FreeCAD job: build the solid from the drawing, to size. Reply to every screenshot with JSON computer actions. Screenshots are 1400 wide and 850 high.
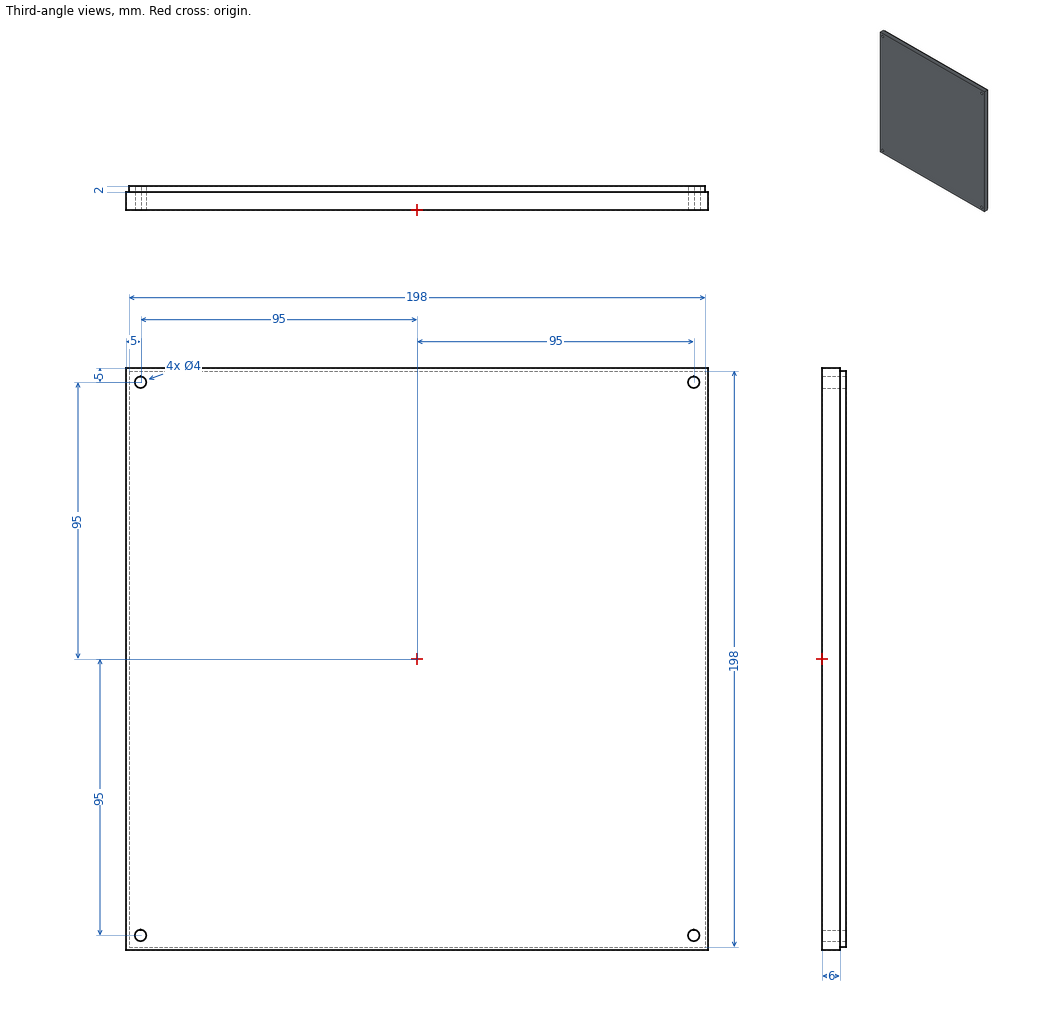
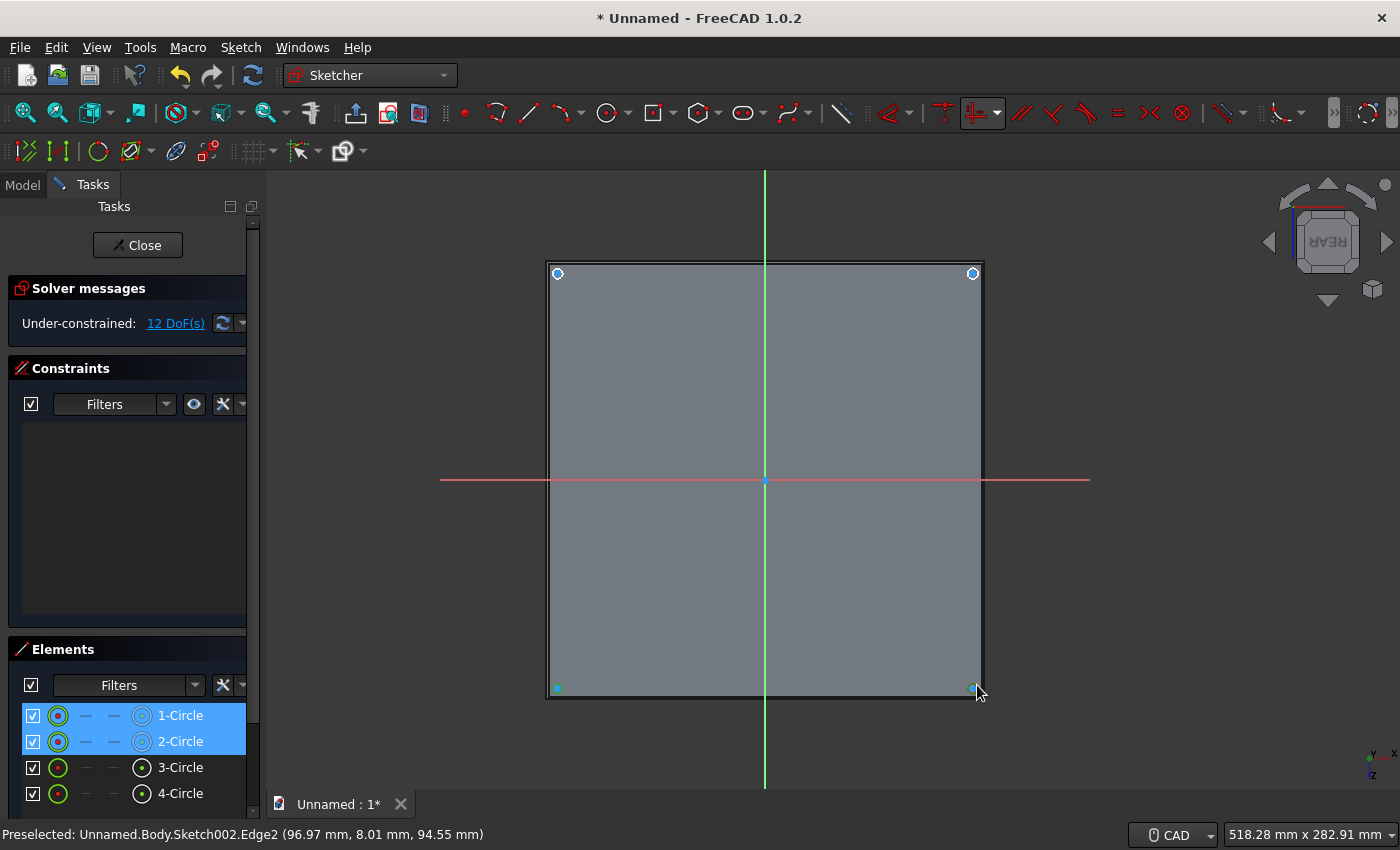
{"action": "scroll", "coordinate": [977, 270], "scroll_direction": "up", "scroll_amount": 5}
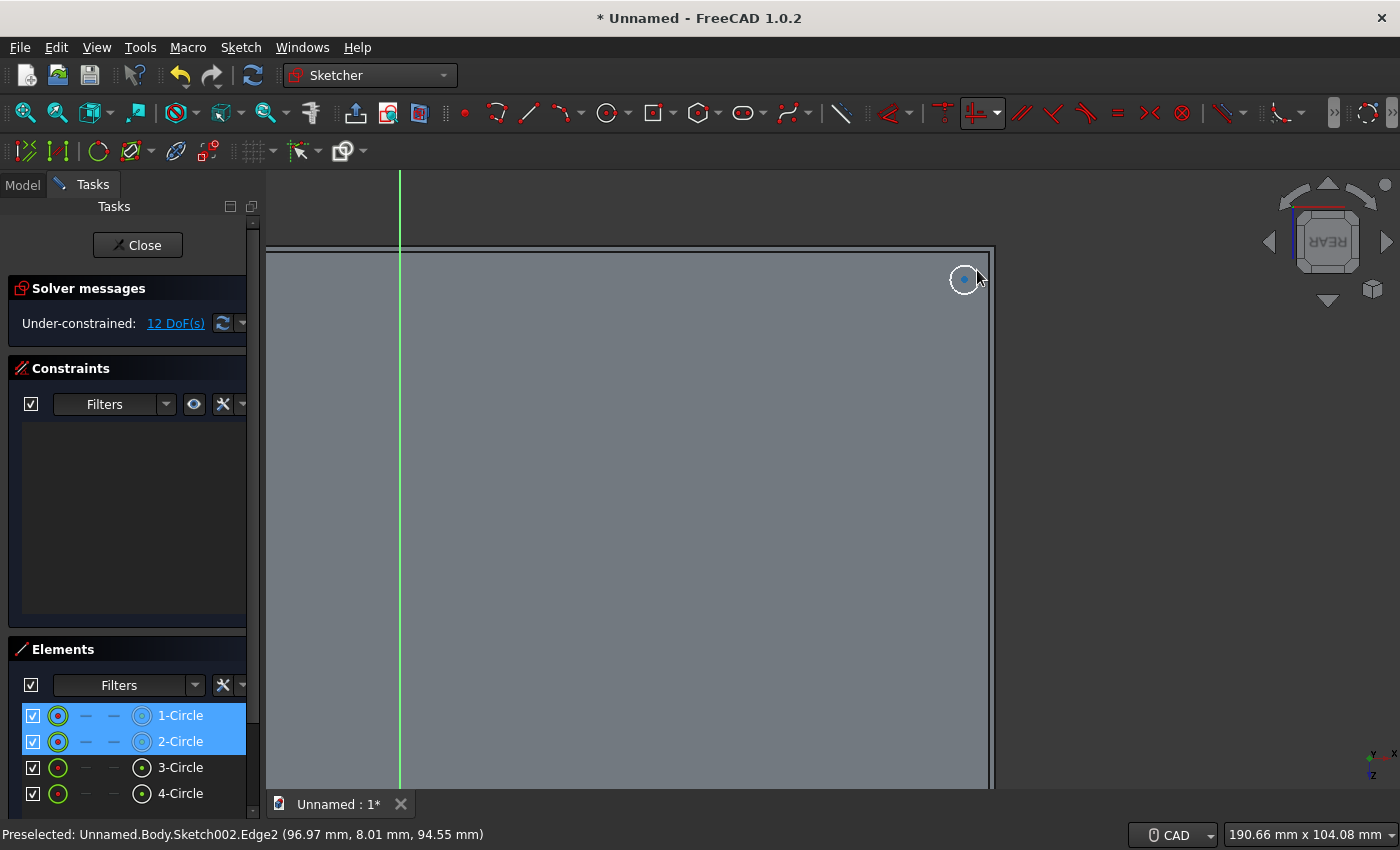
{"action": "left_click", "coordinate": [975, 270]}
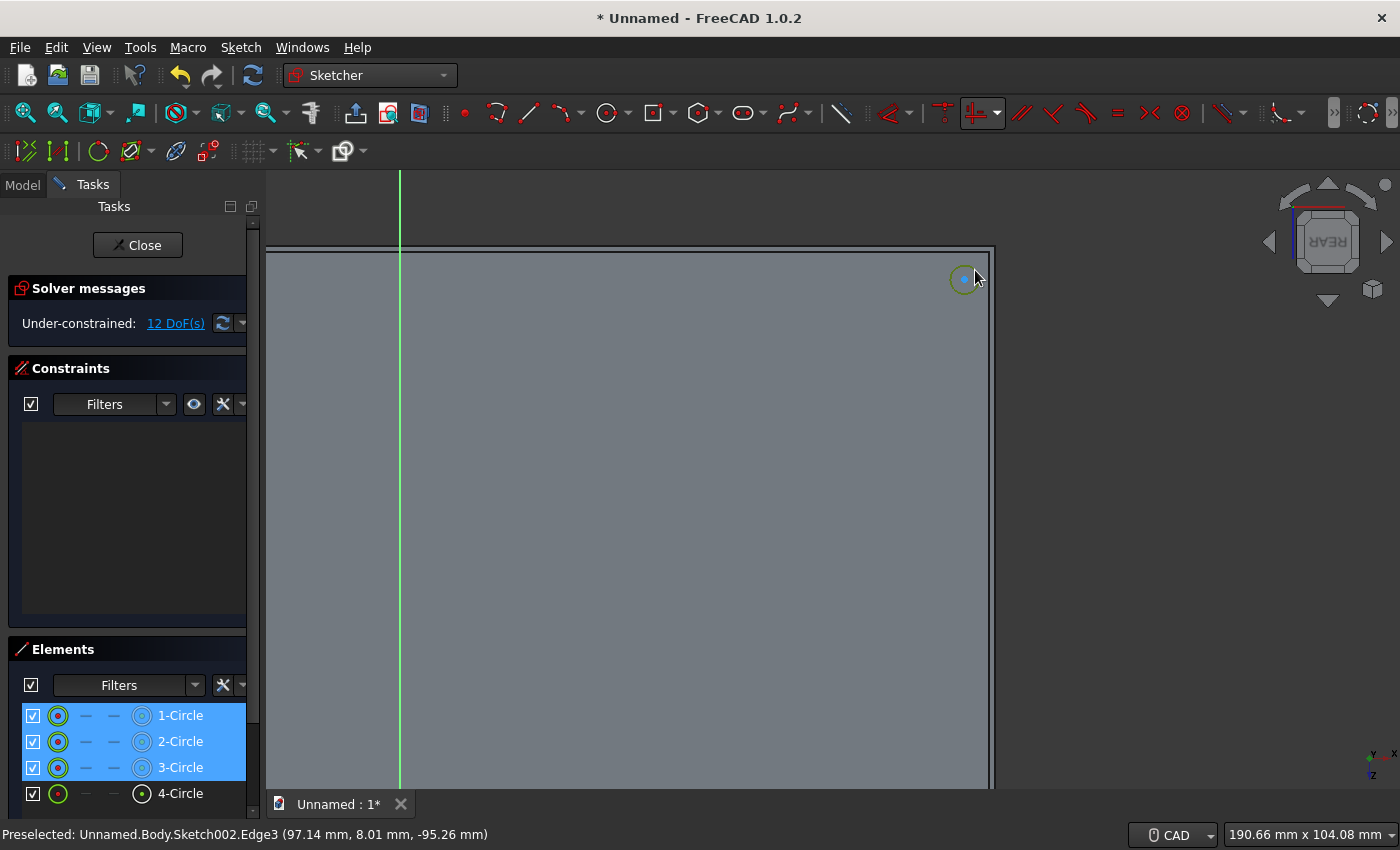
{"action": "scroll", "coordinate": [977, 269], "scroll_direction": "down", "scroll_amount": 5}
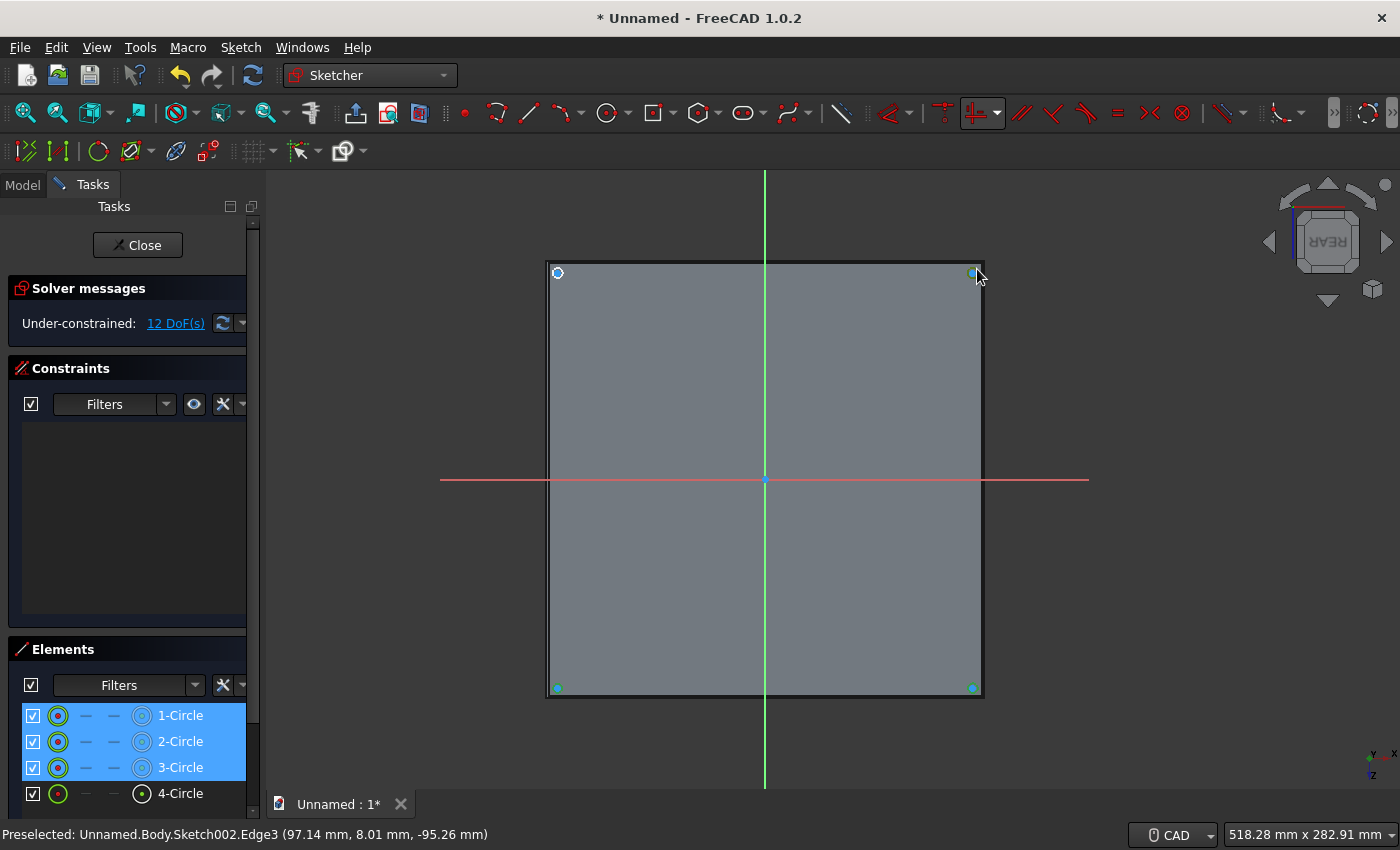
{"action": "scroll", "coordinate": [561, 270], "scroll_direction": "up", "scroll_amount": 6}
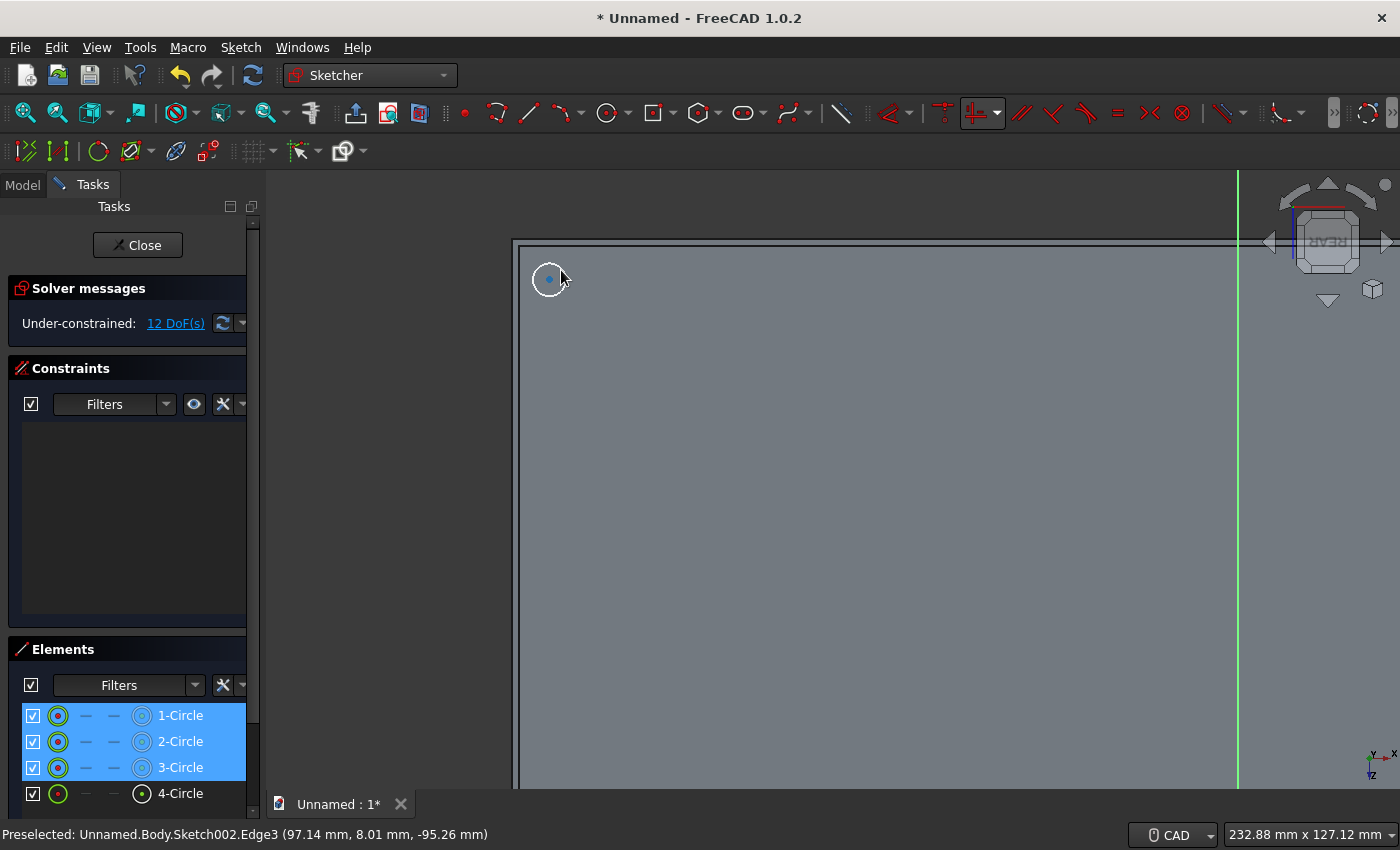
{"action": "left_click", "coordinate": [561, 268]}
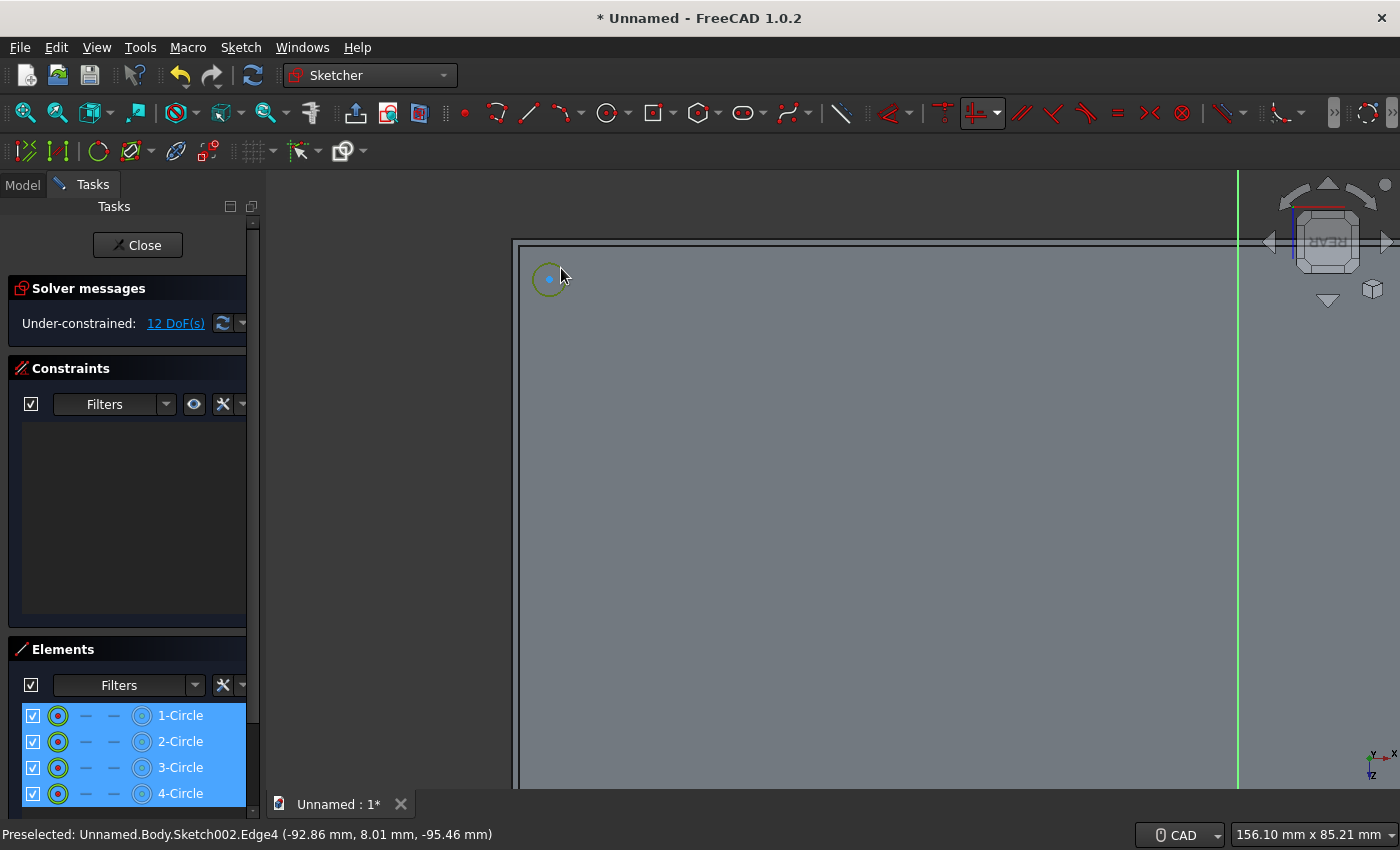
{"action": "key", "text": "e"}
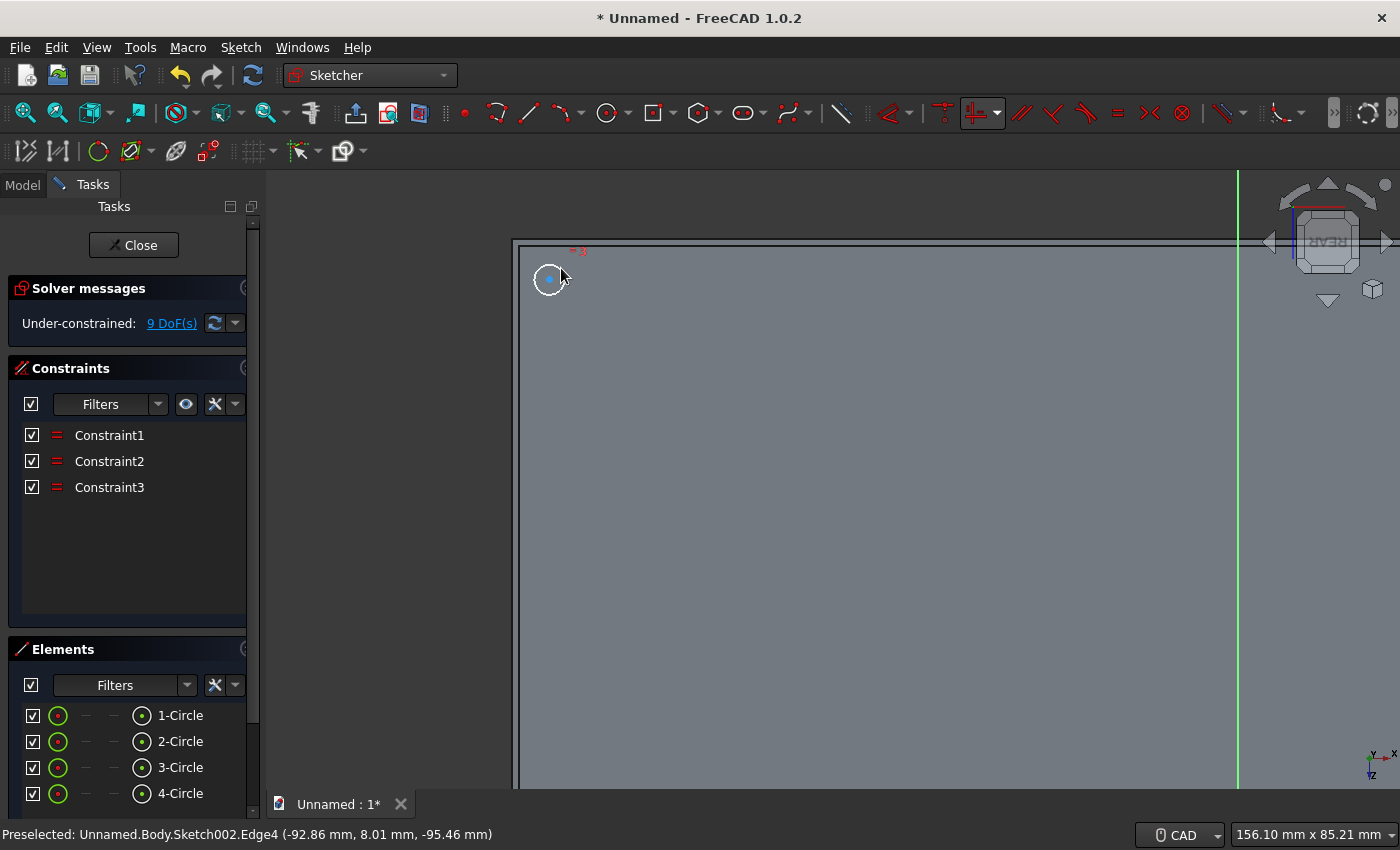
{"action": "scroll", "coordinate": [560, 270], "scroll_direction": "down", "scroll_amount": 6}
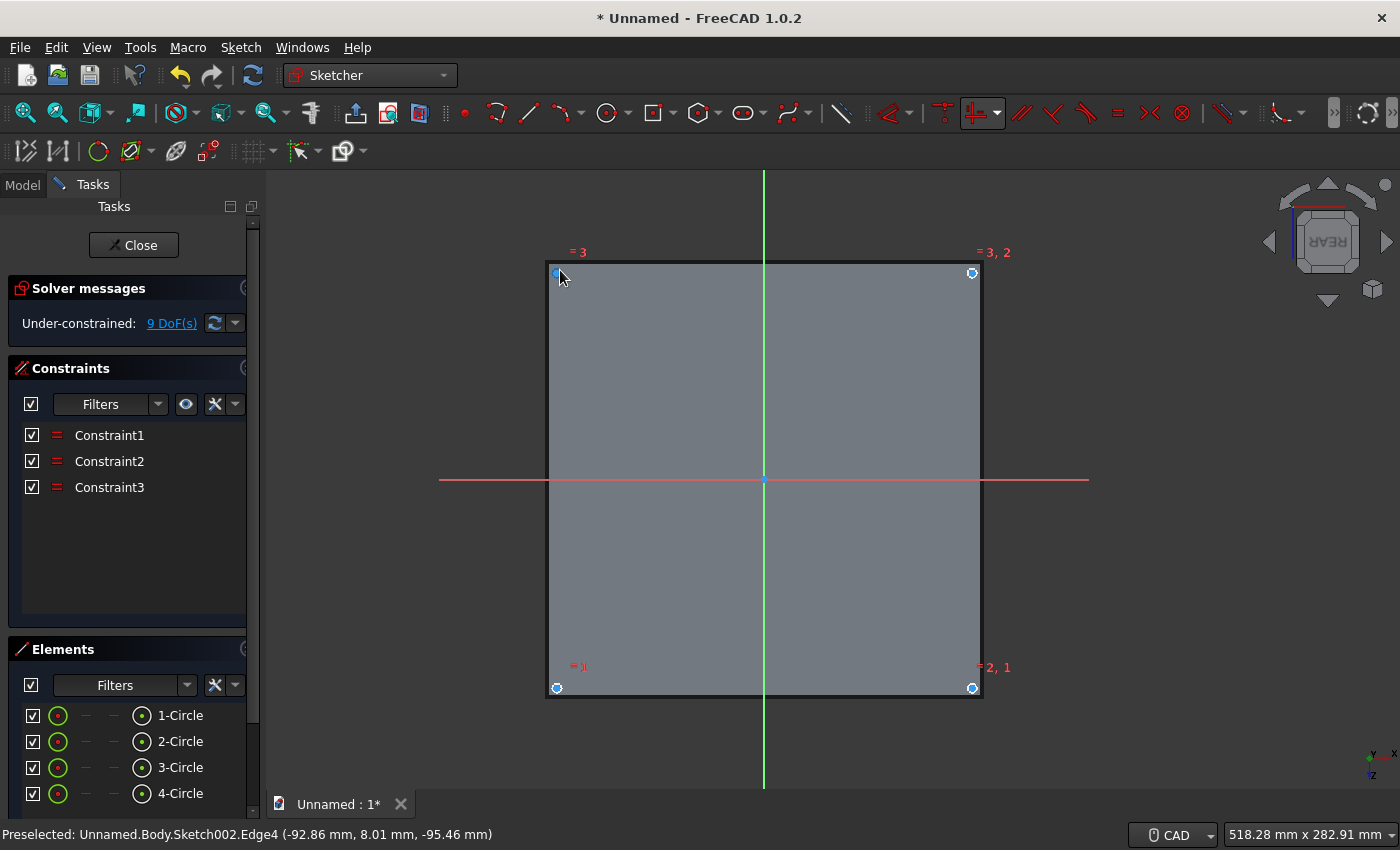
{"action": "left_click", "coordinate": [557, 688]}